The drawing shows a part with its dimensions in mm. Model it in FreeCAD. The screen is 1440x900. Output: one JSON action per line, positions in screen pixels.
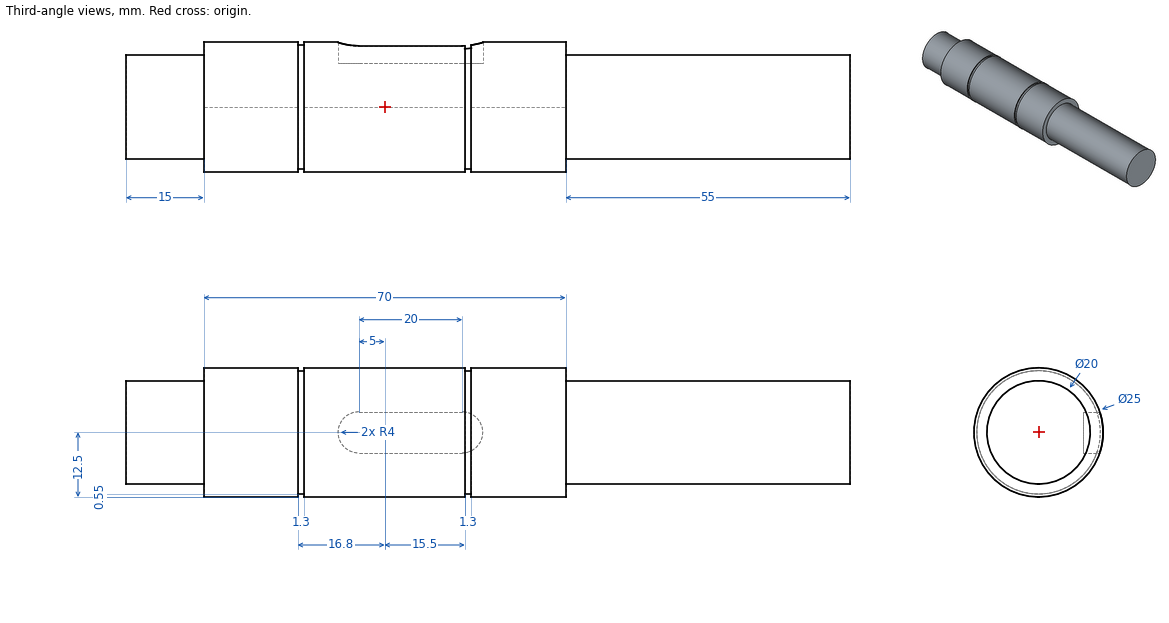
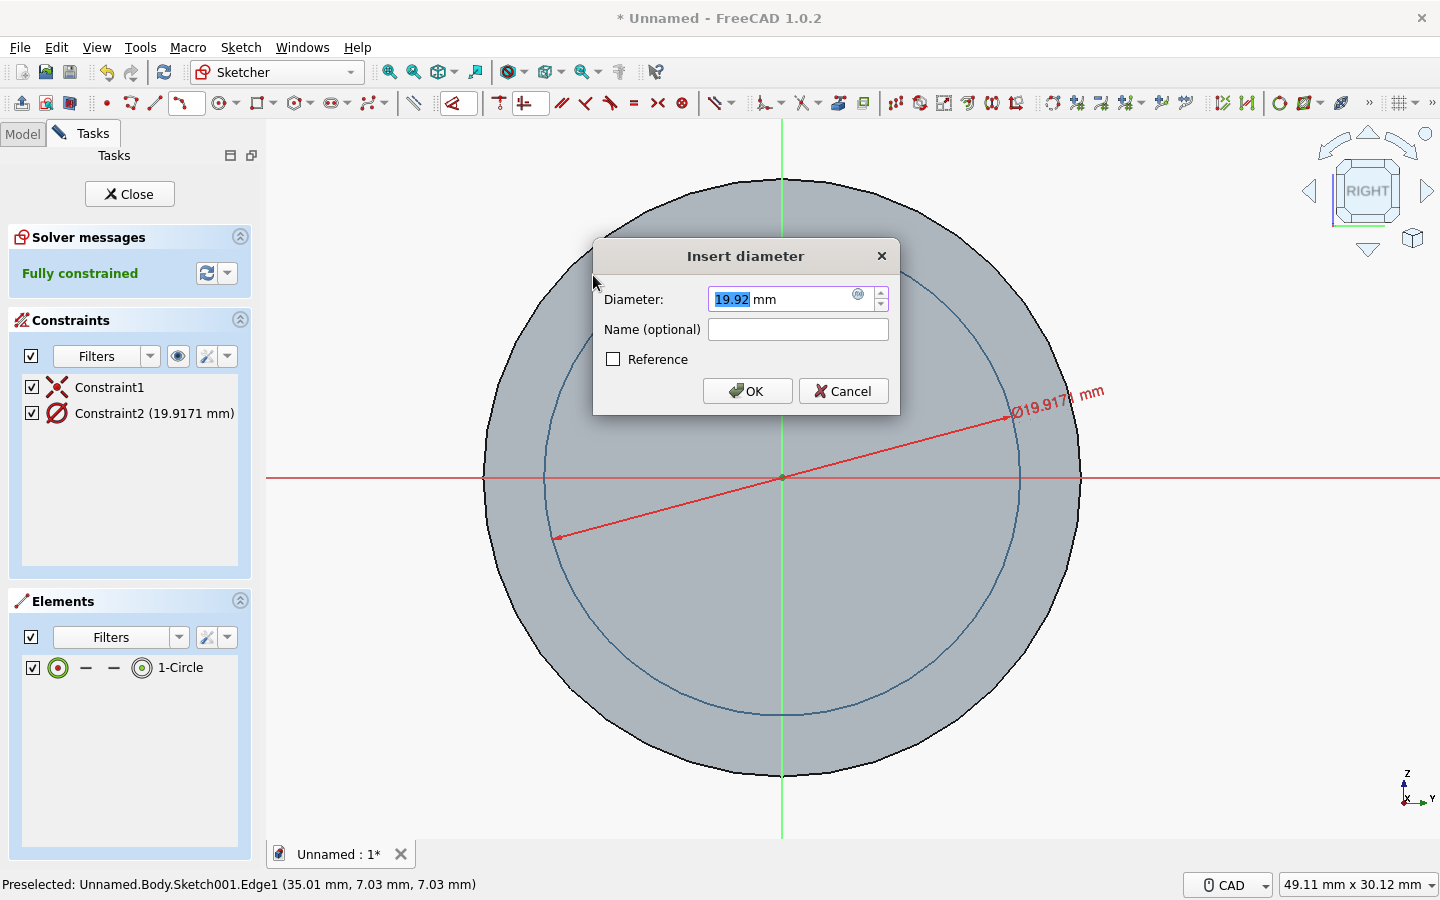
{"action": "type", "text": "20"}
{"action": "key", "text": "Return"}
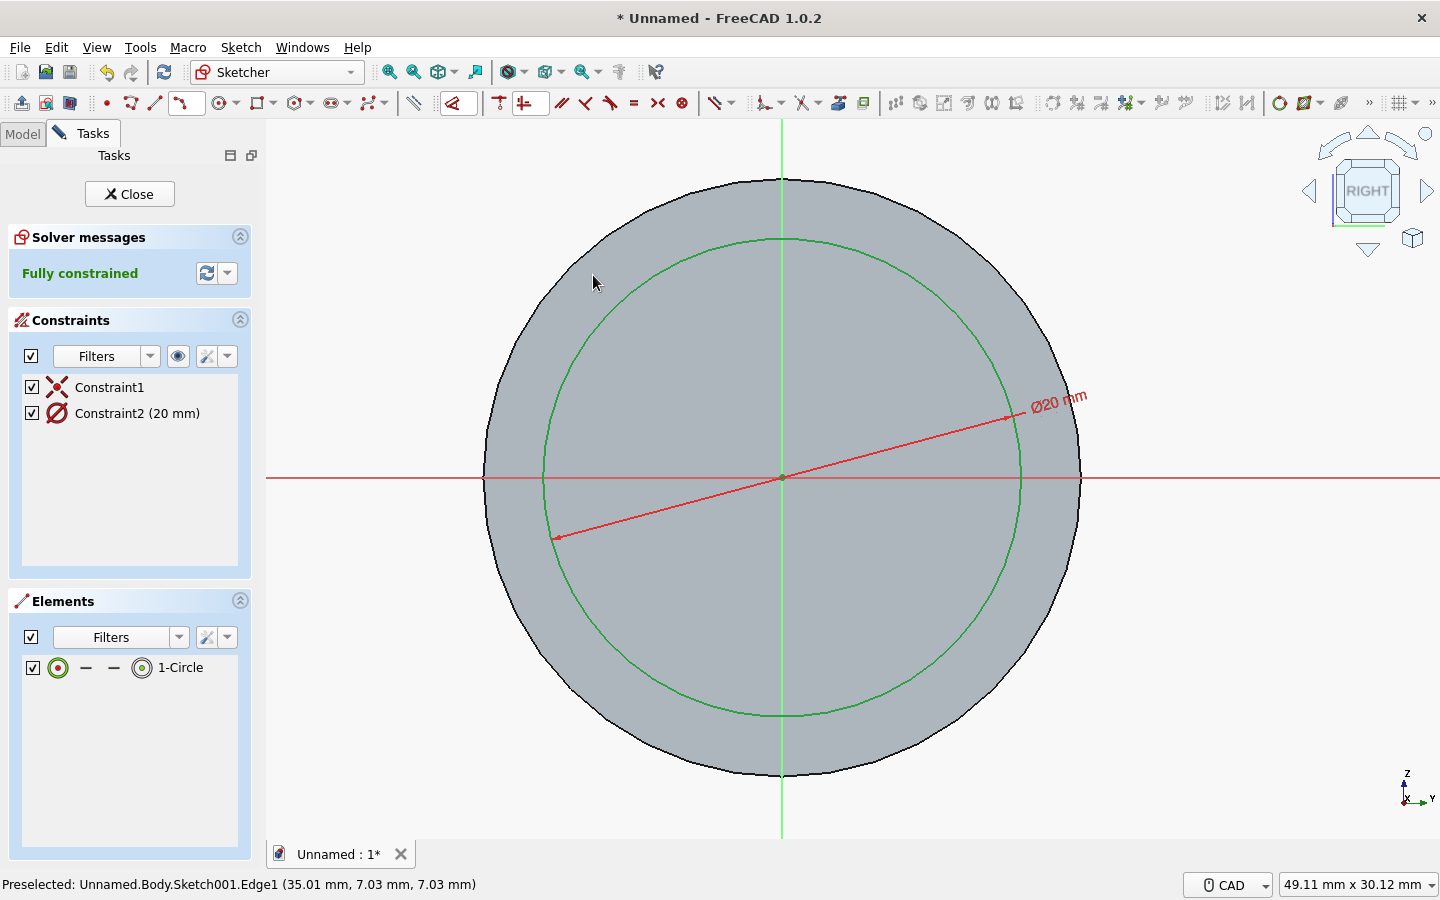
{"action": "left_click", "coordinate": [130, 194]}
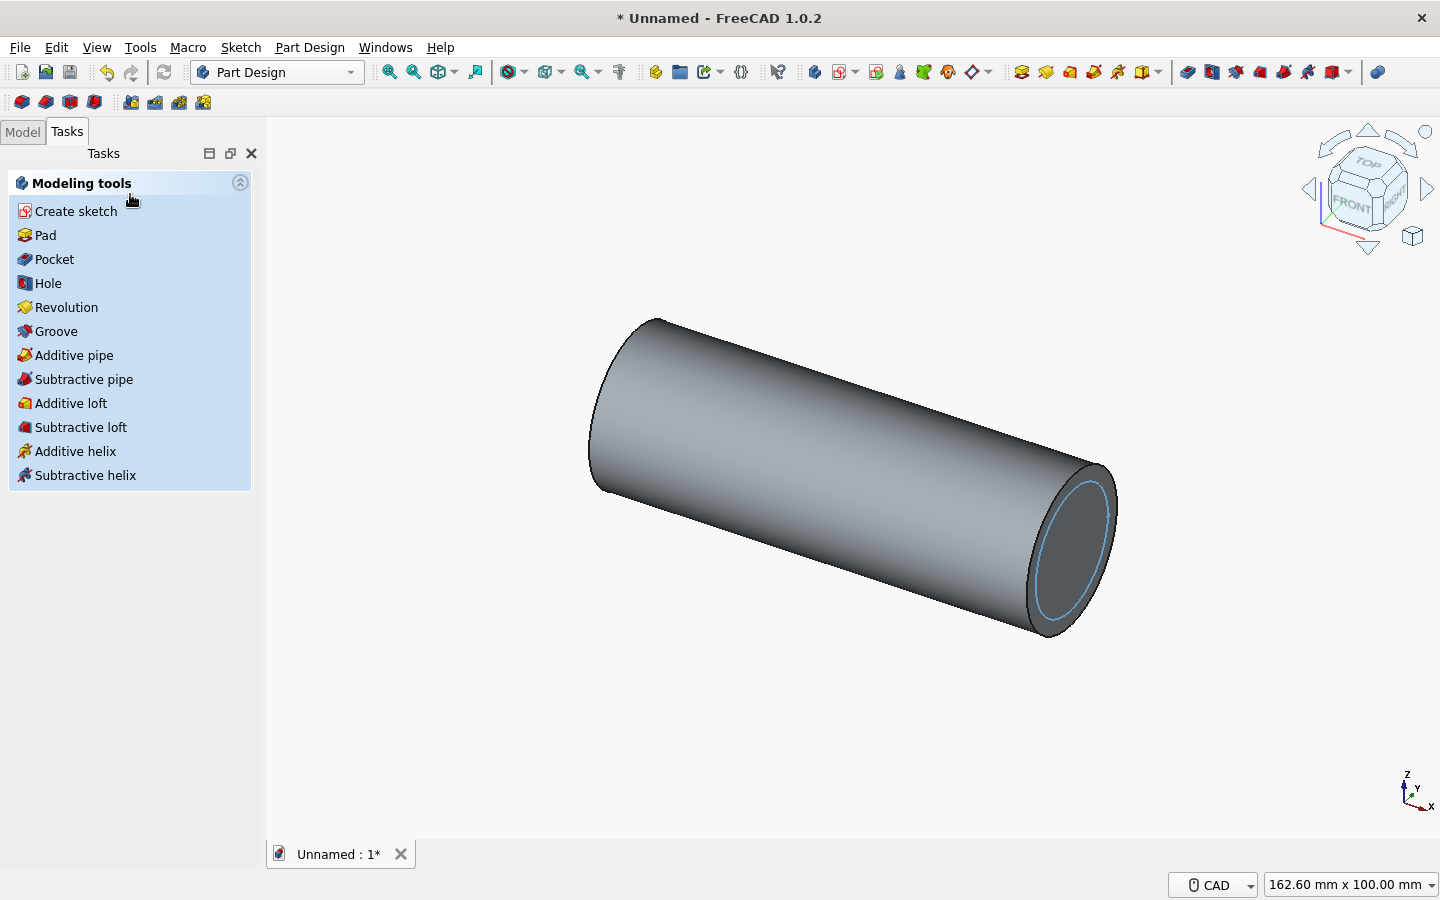
{"action": "left_click", "coordinate": [1022, 72]}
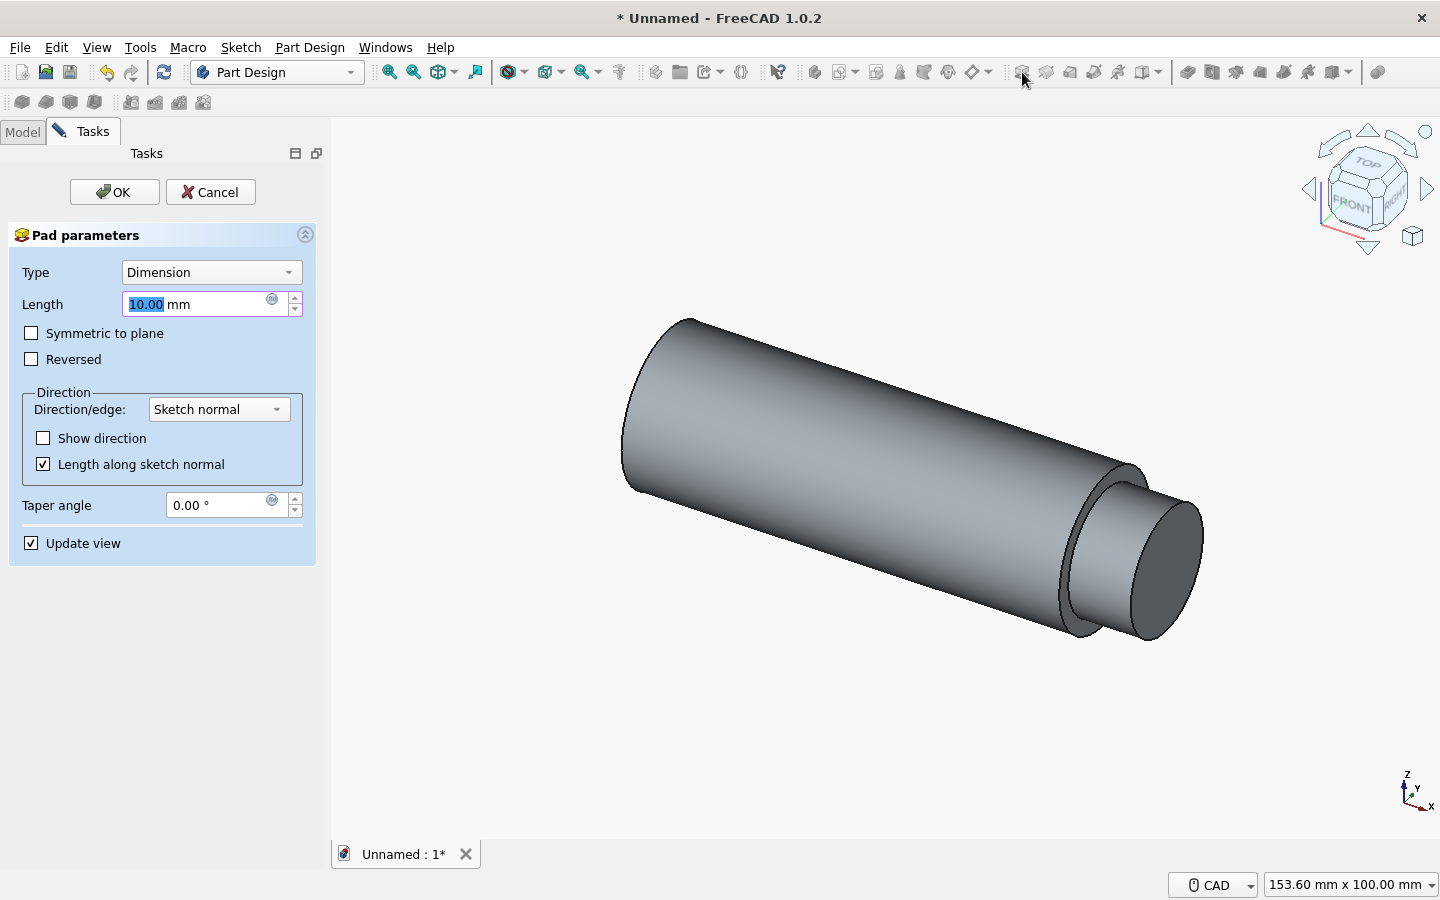
{"action": "type", "text": "55"}
{"action": "key", "text": "Tab"}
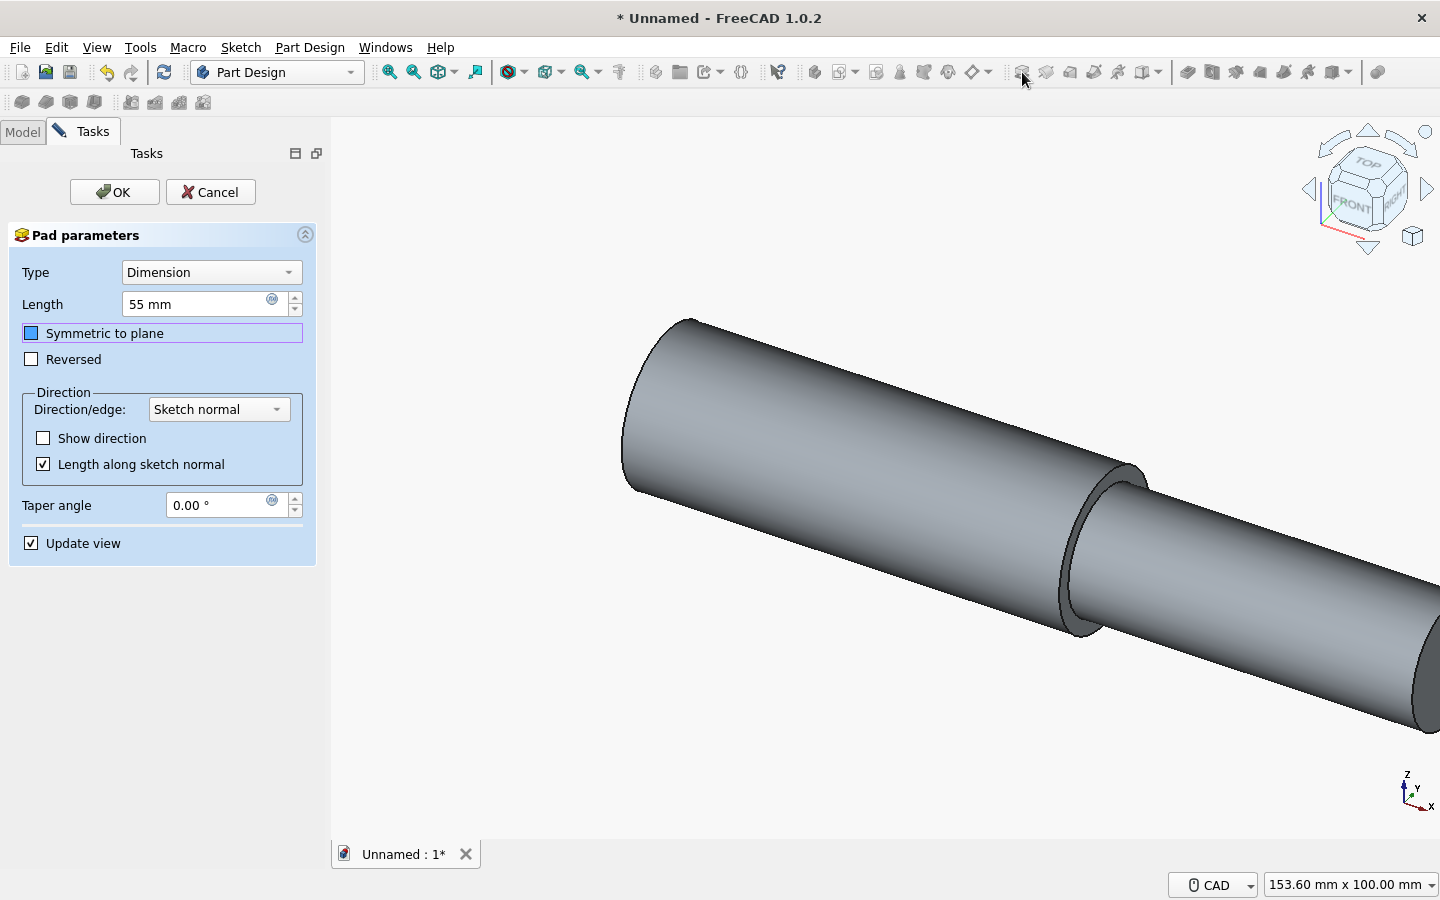
{"action": "left_click", "coordinate": [115, 192]}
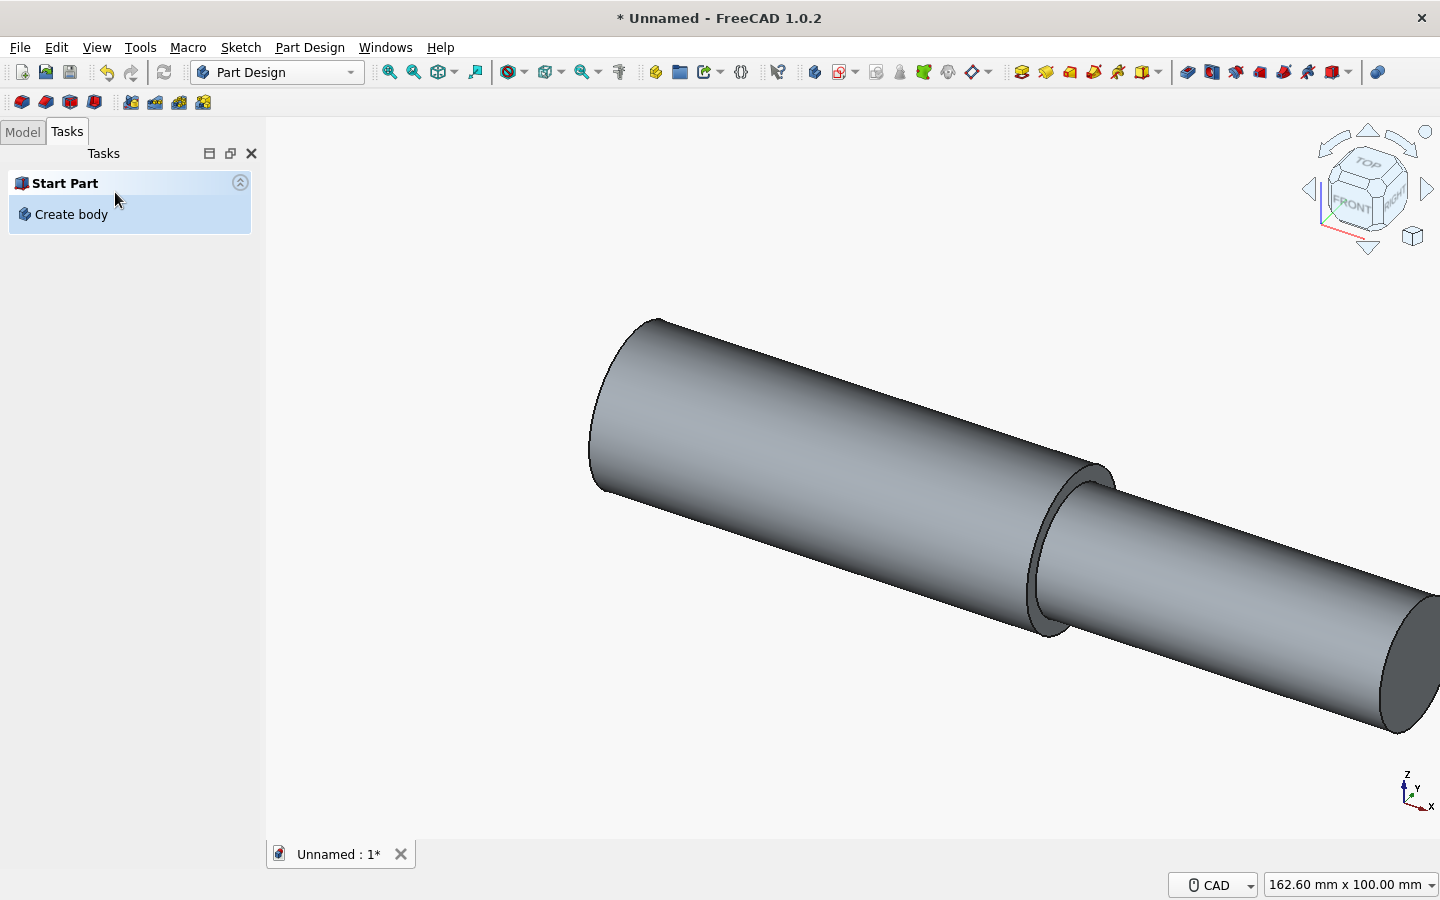
{"action": "left_click", "coordinate": [390, 72]}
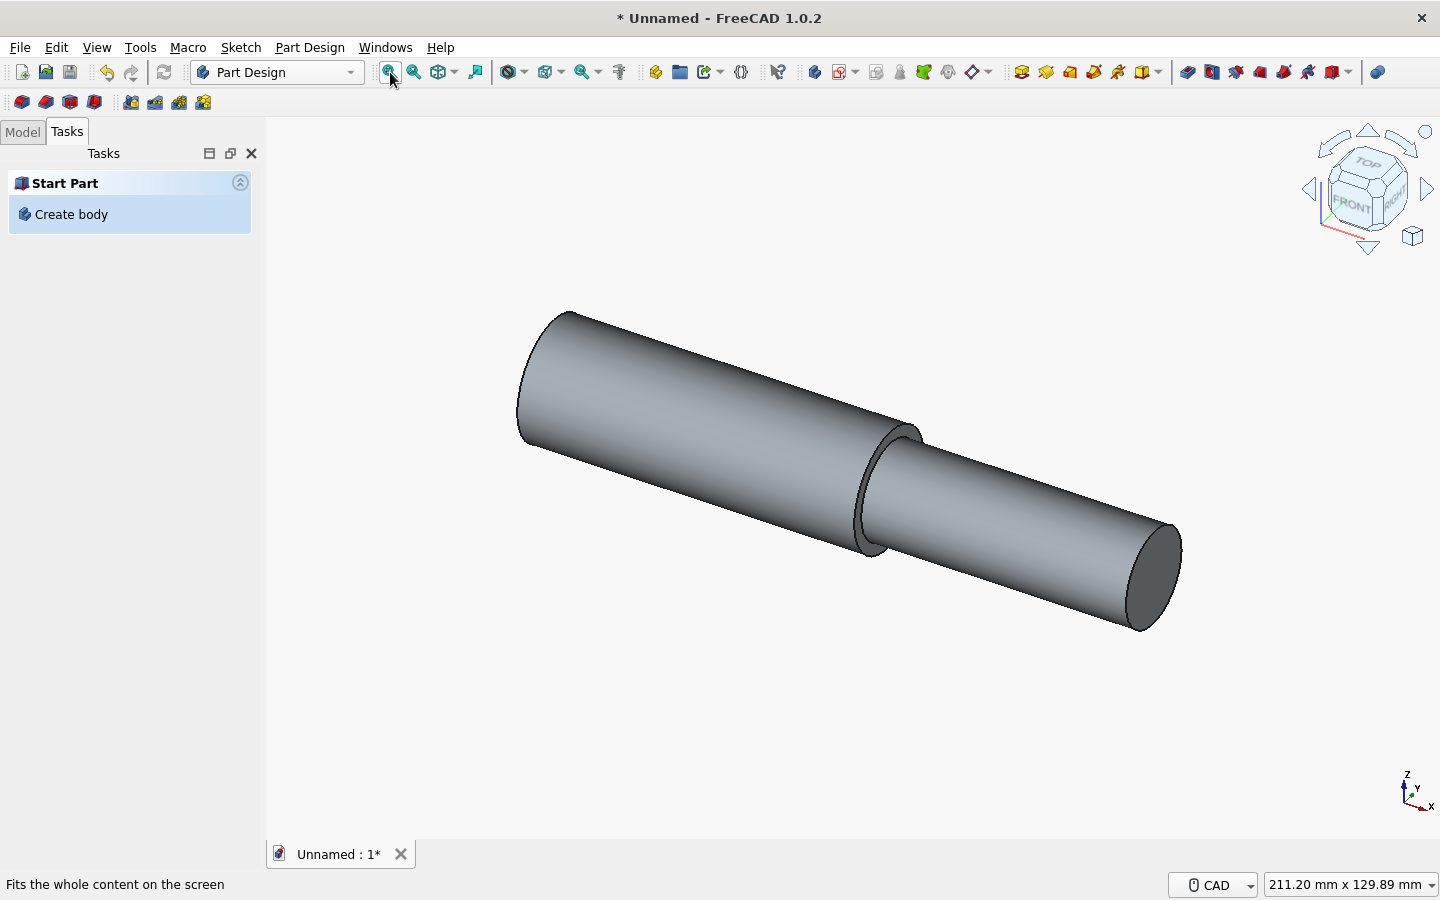
{"action": "left_click", "coordinate": [840, 72]}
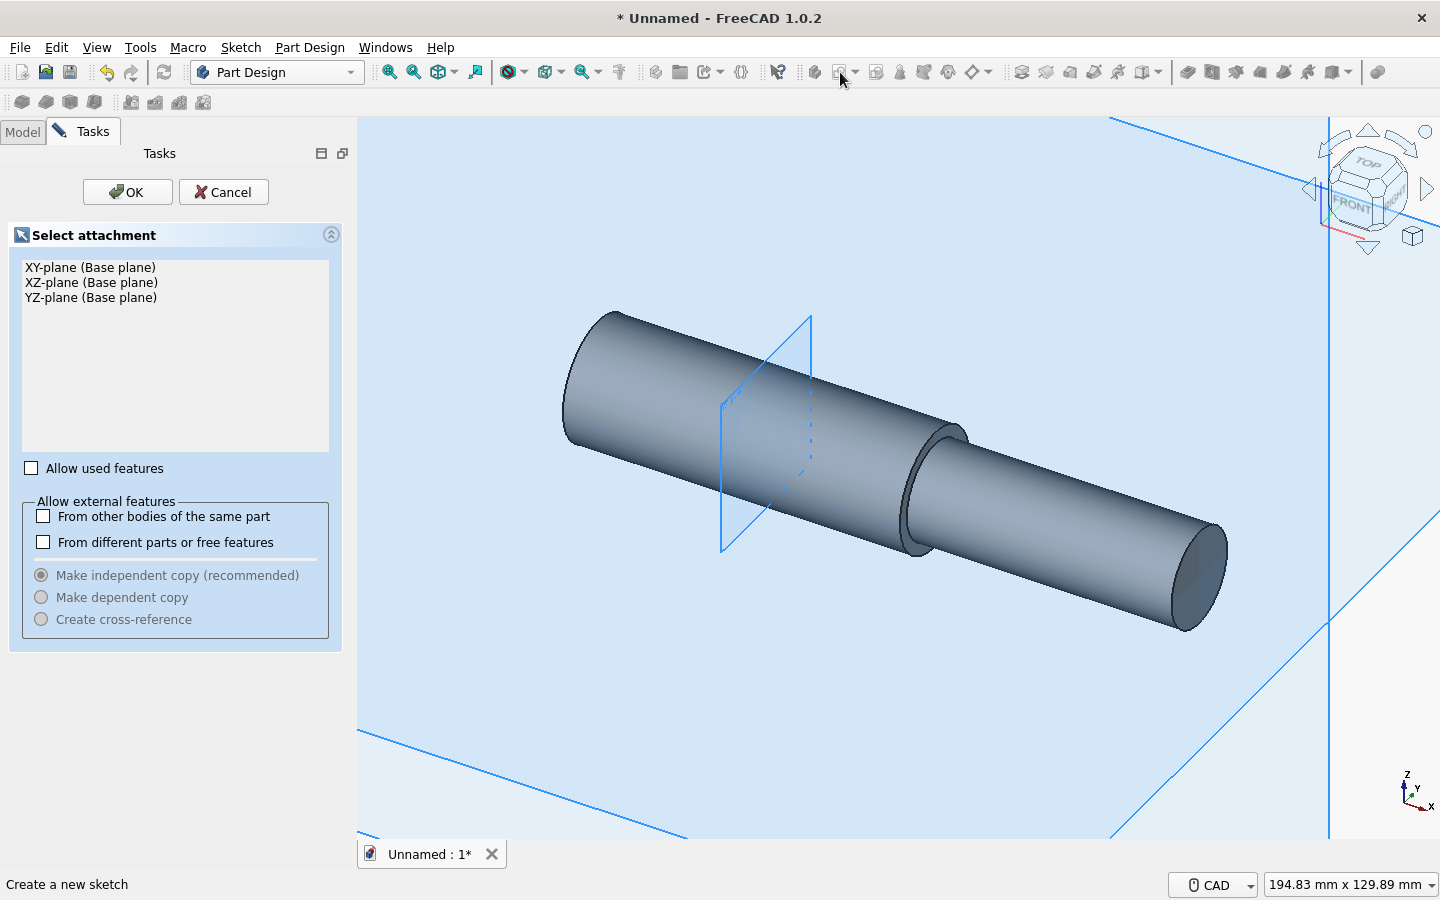
{"action": "left_click", "coordinate": [82, 282]}